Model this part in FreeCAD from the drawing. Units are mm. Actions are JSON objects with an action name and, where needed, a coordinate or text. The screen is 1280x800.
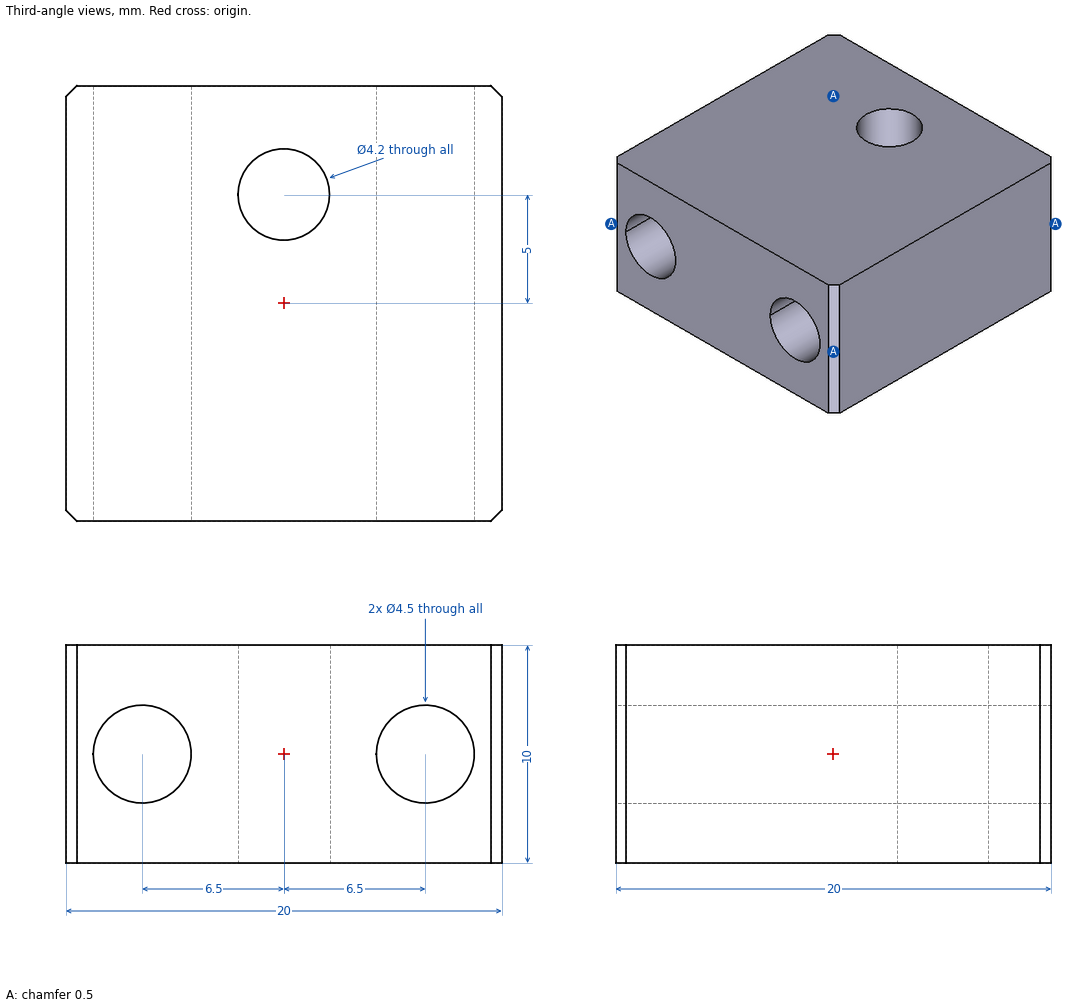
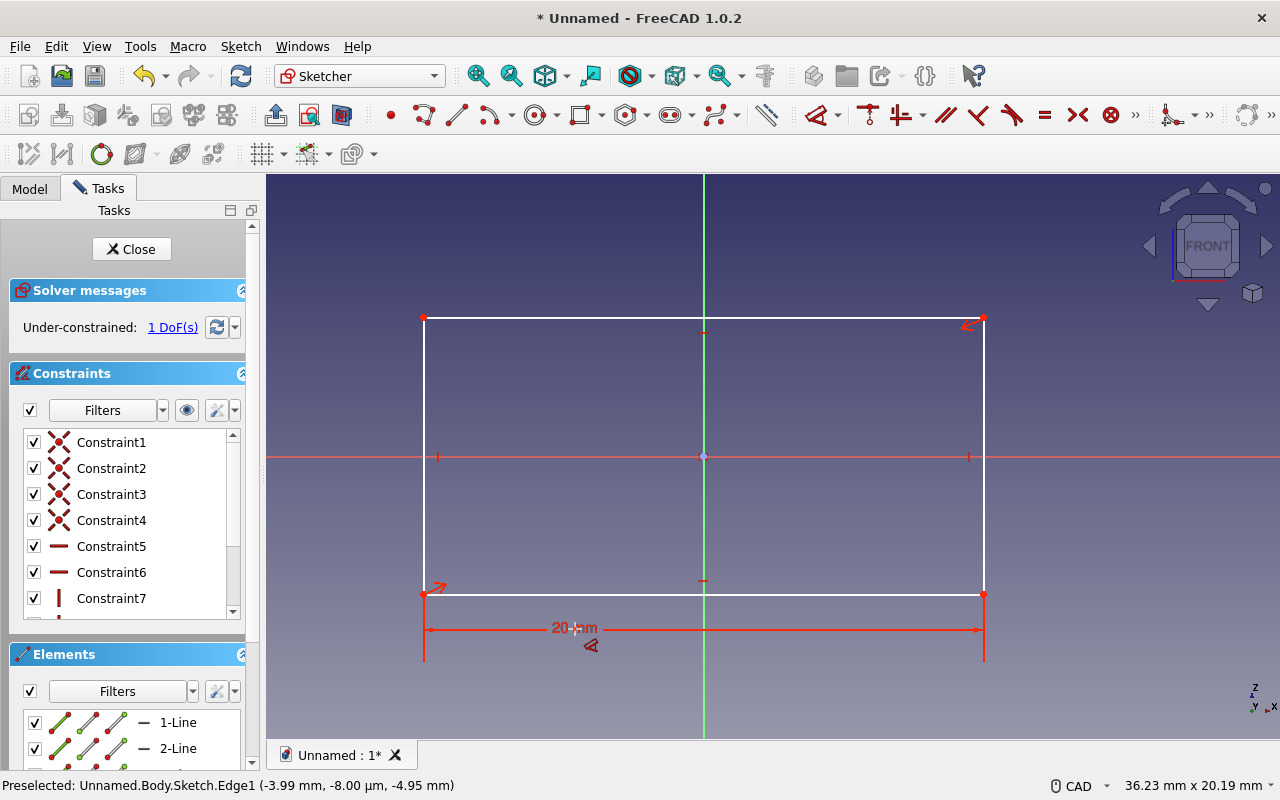
{"action": "left_click", "coordinate": [984, 512]}
{"action": "left_click", "coordinate": [1018, 393]}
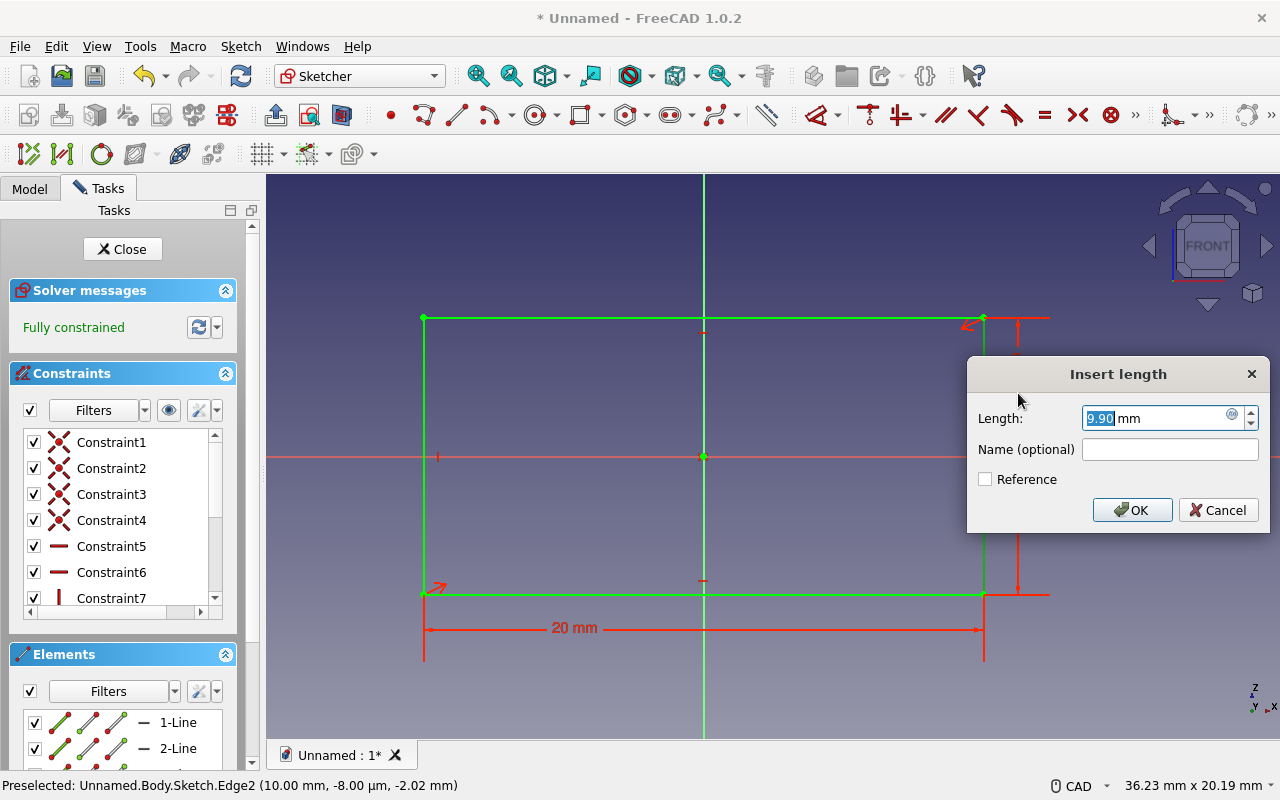
{"action": "type", "text": "10"}
{"action": "key", "text": "Return"}
{"action": "key", "text": "Escape"}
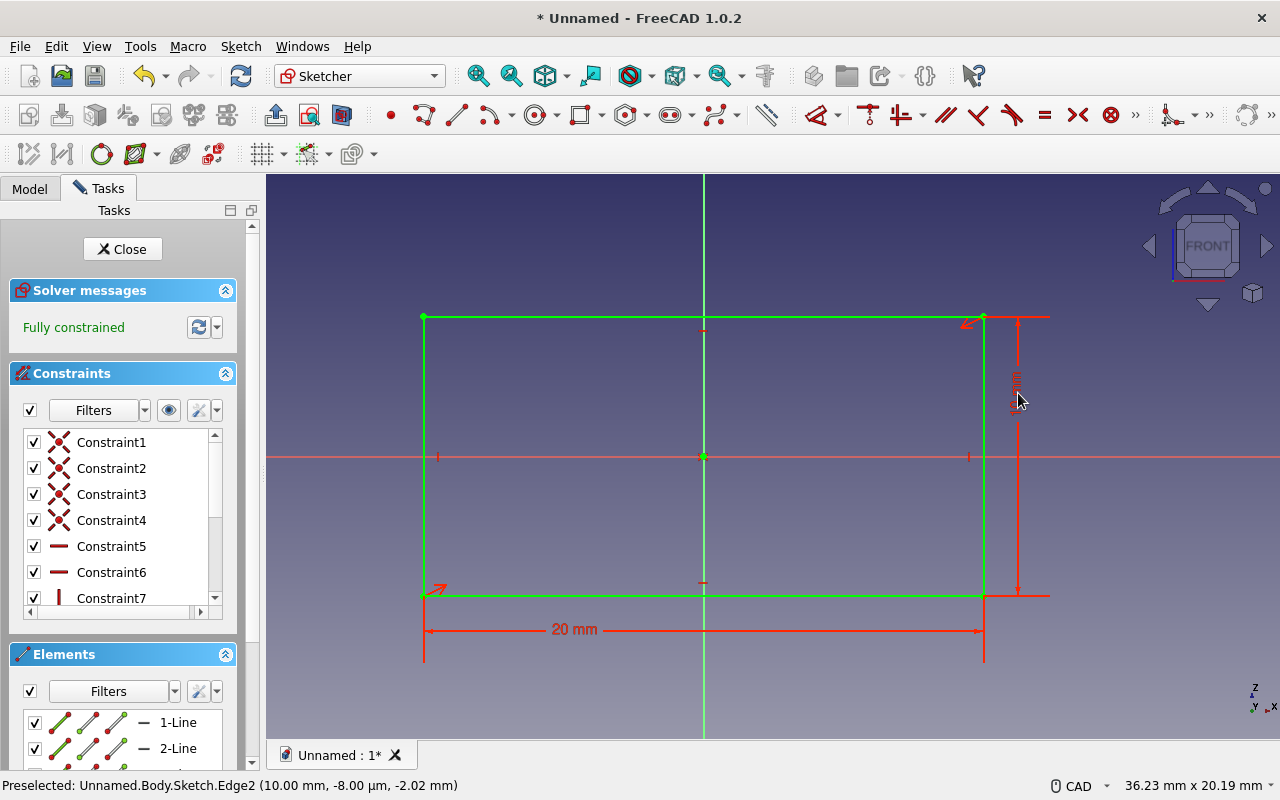
{"action": "left_click", "coordinate": [123, 249]}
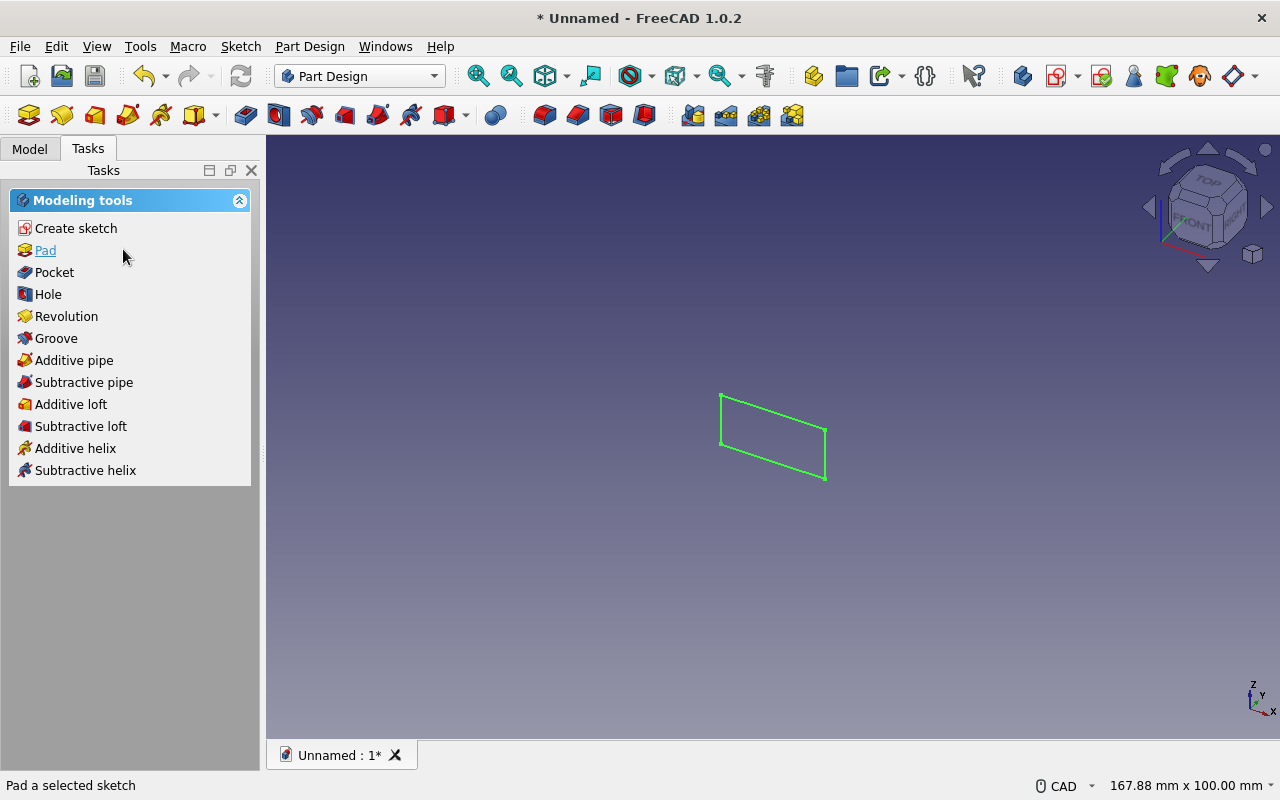
{"action": "left_click", "coordinate": [29, 116]}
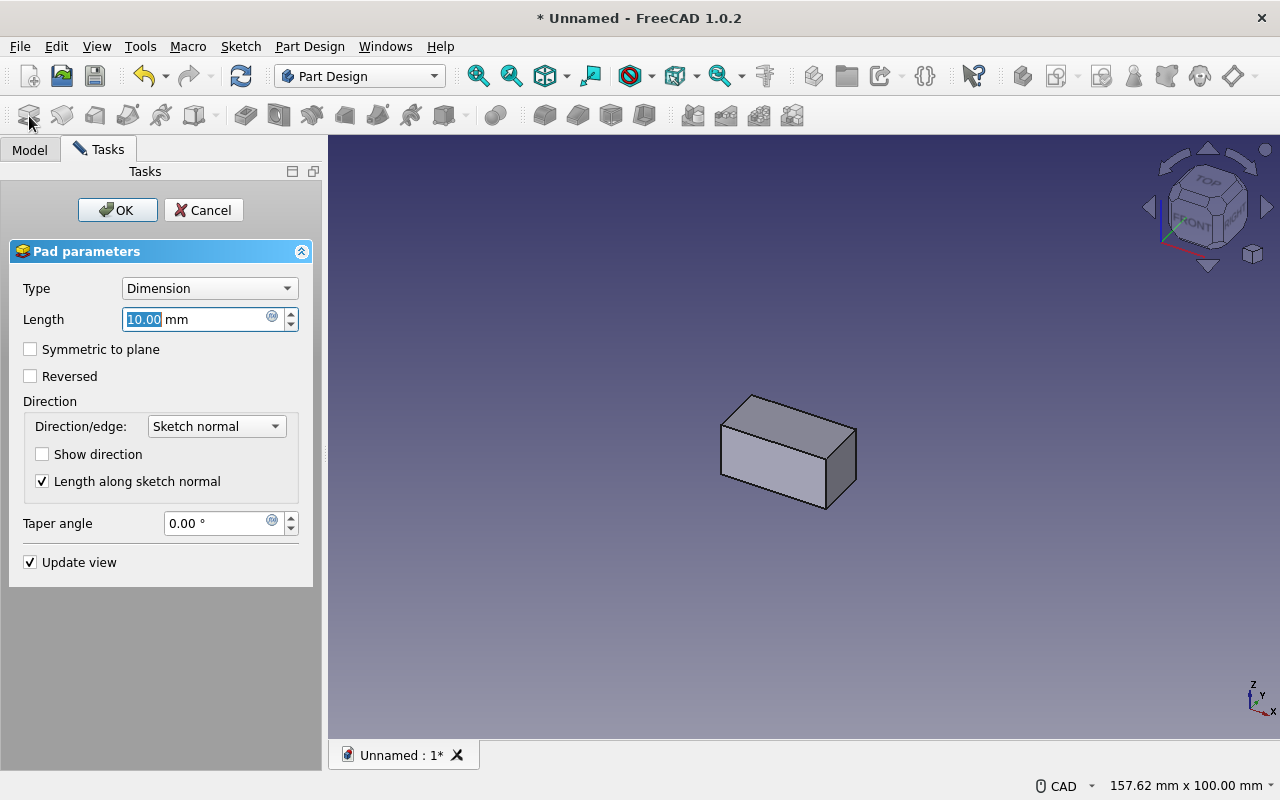
{"action": "type", "text": "20"}
{"action": "key", "text": "Tab"}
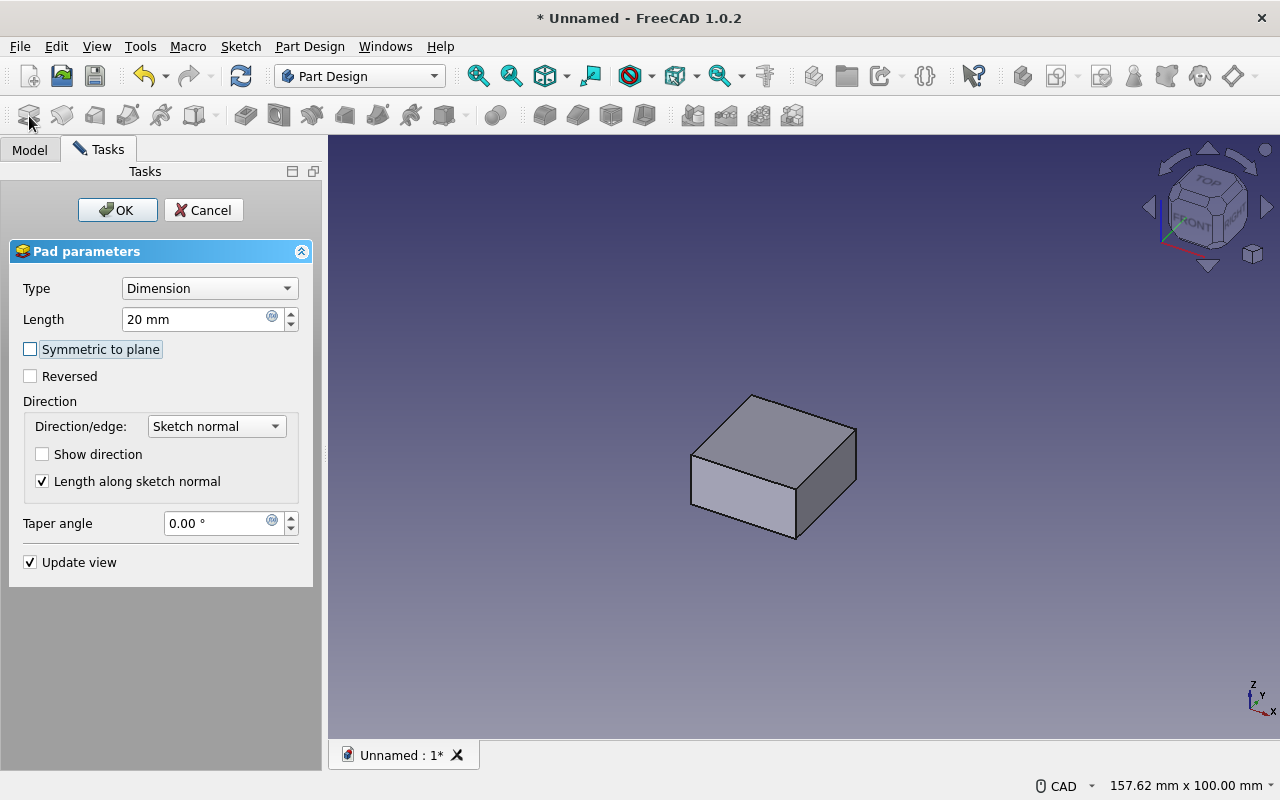
{"action": "left_click", "coordinate": [31, 349]}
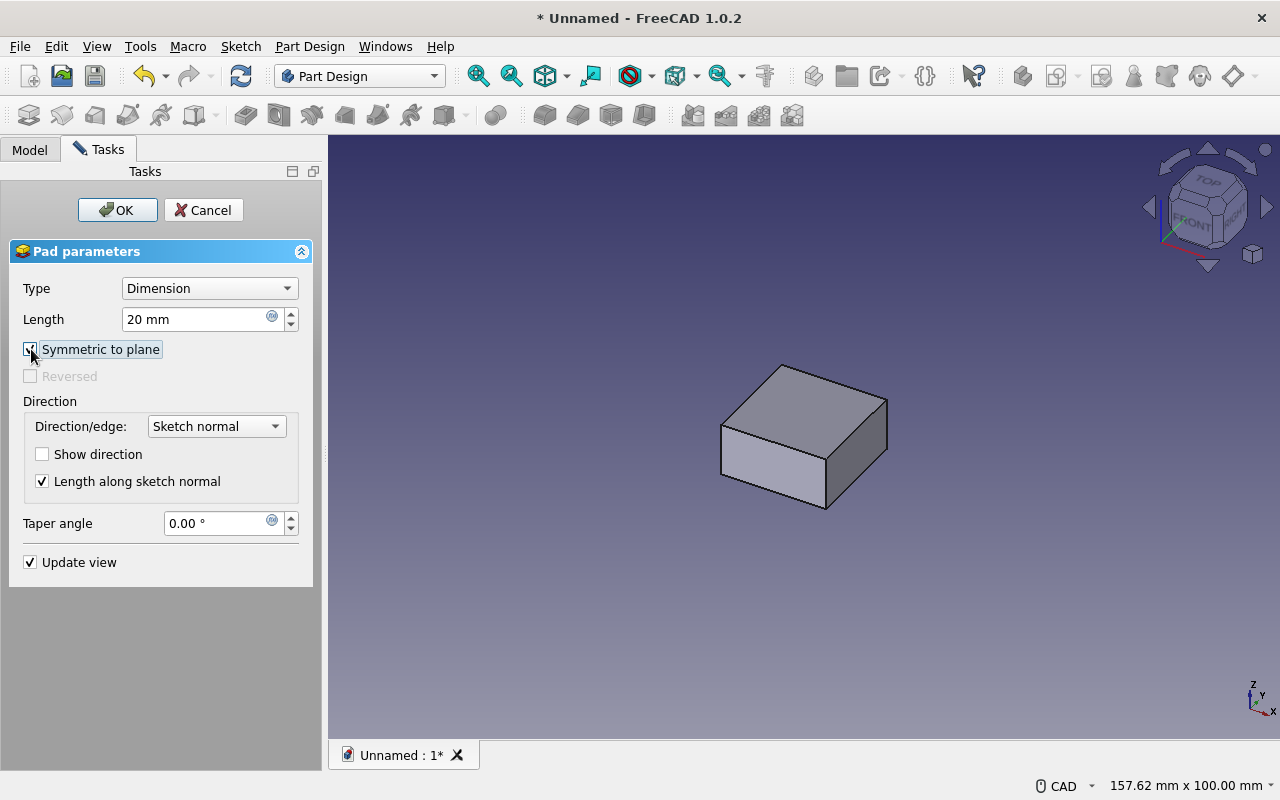
{"action": "left_click", "coordinate": [118, 210]}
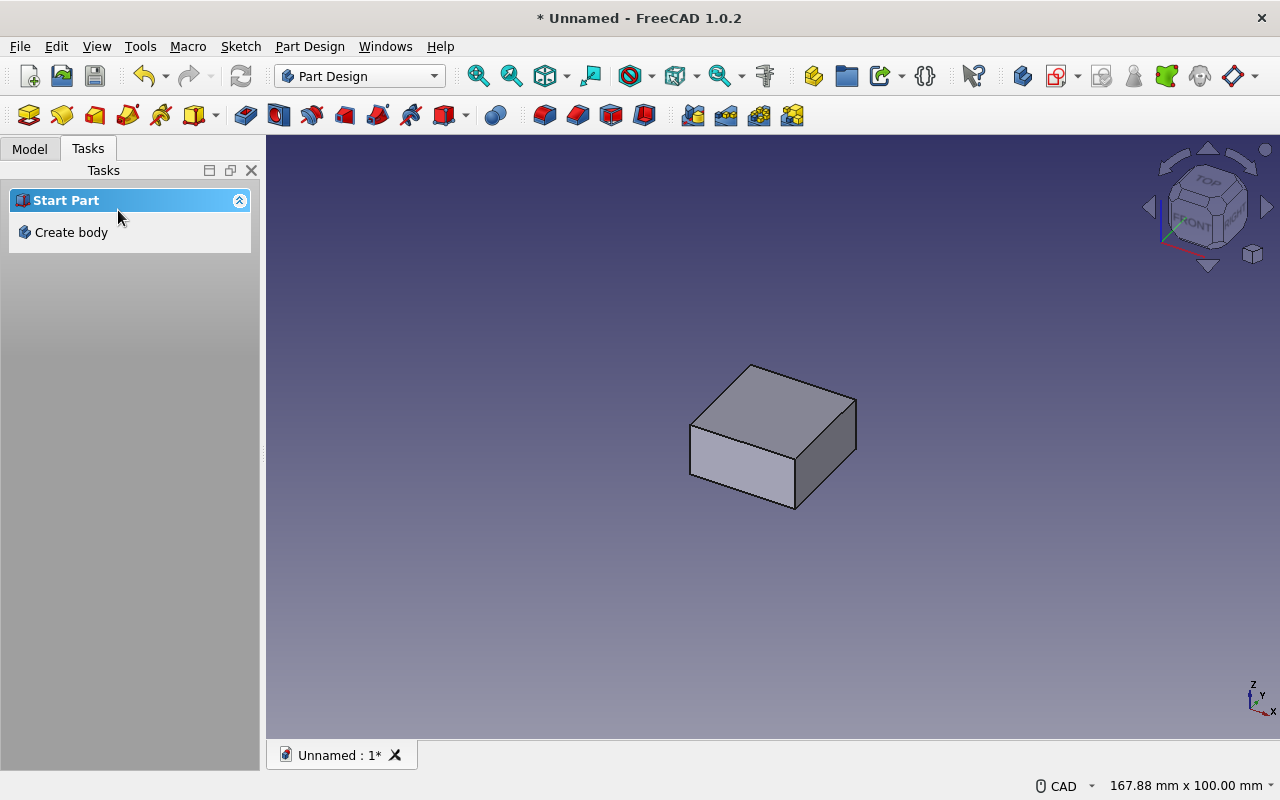
{"action": "key", "text": "v f"}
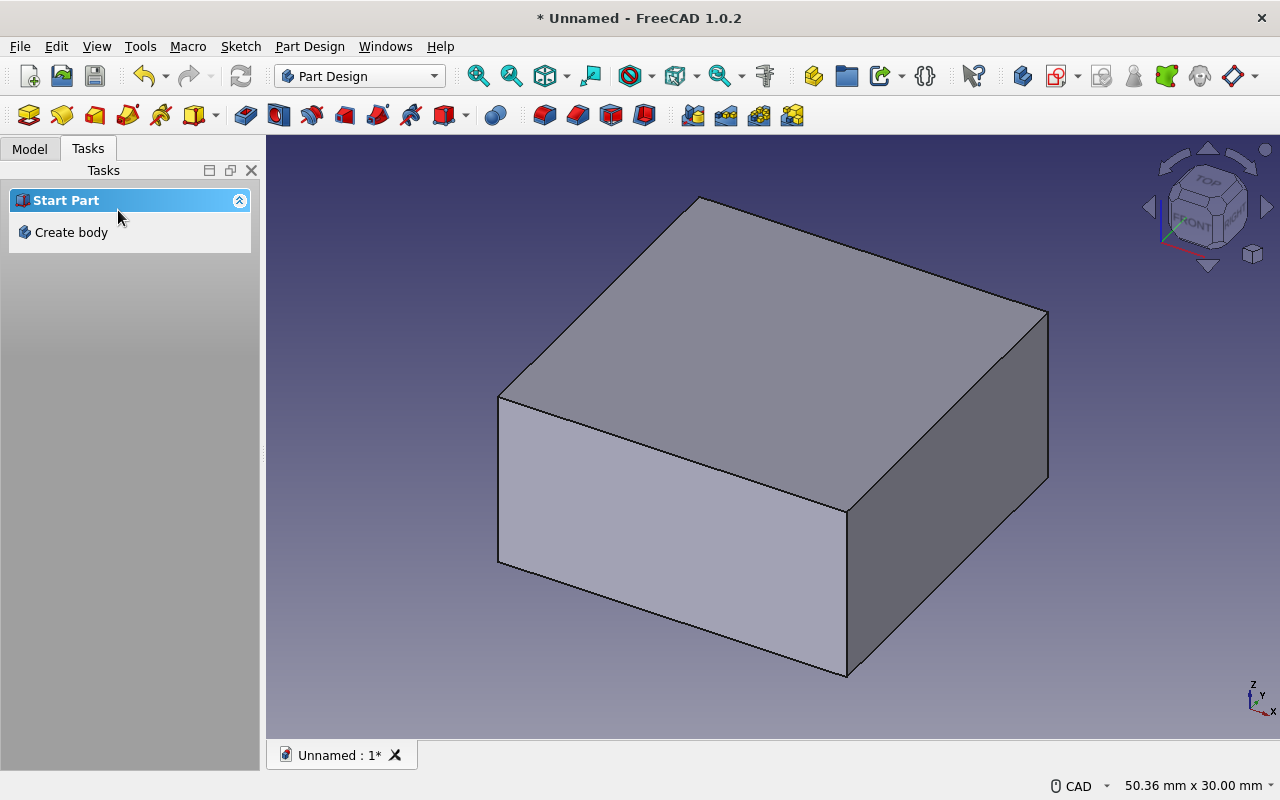
{"action": "left_click", "coordinate": [773, 354]}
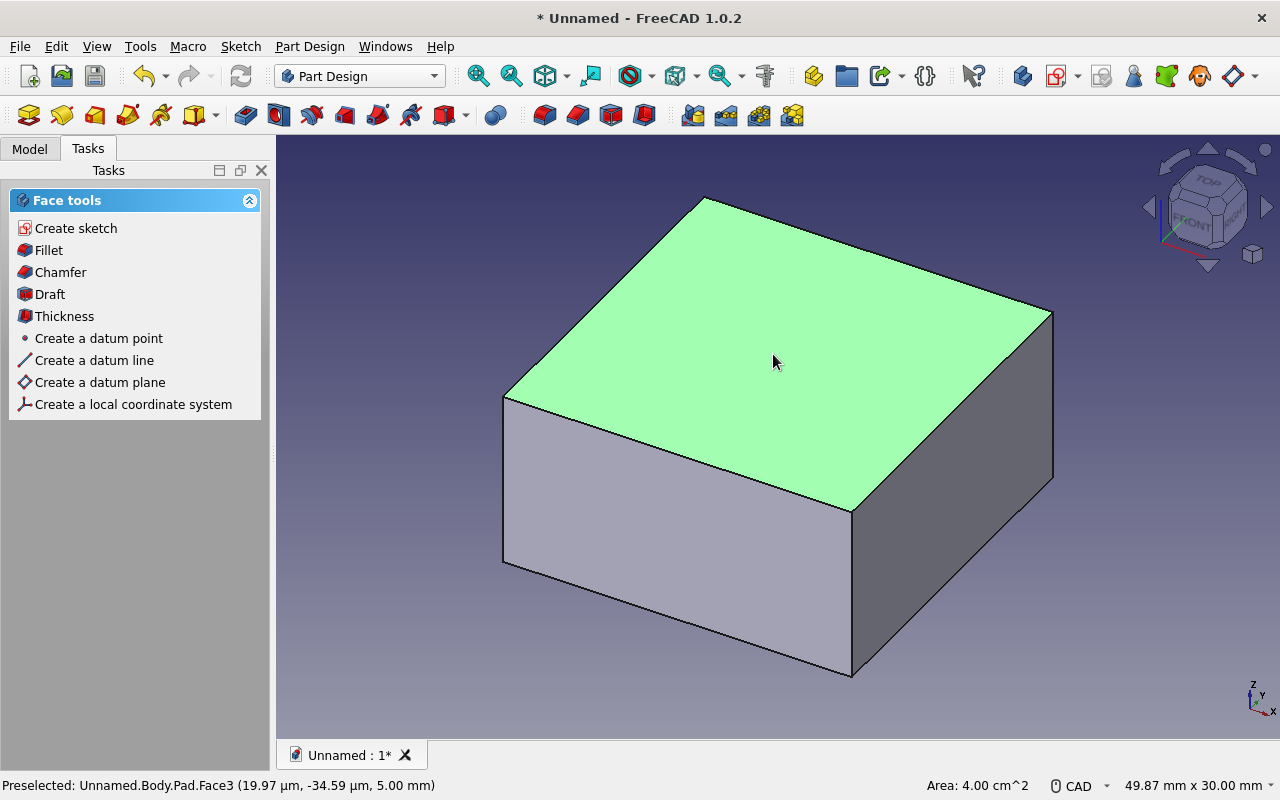
{"action": "left_click", "coordinate": [1056, 76]}